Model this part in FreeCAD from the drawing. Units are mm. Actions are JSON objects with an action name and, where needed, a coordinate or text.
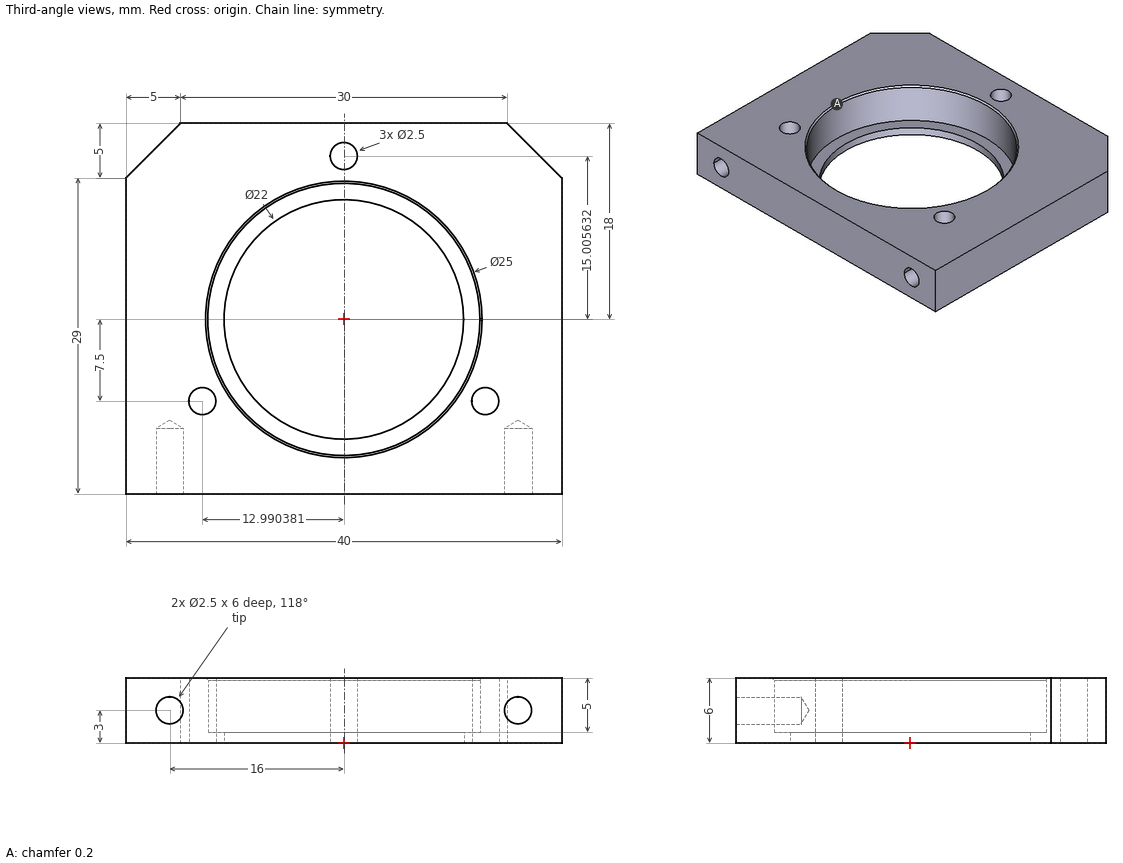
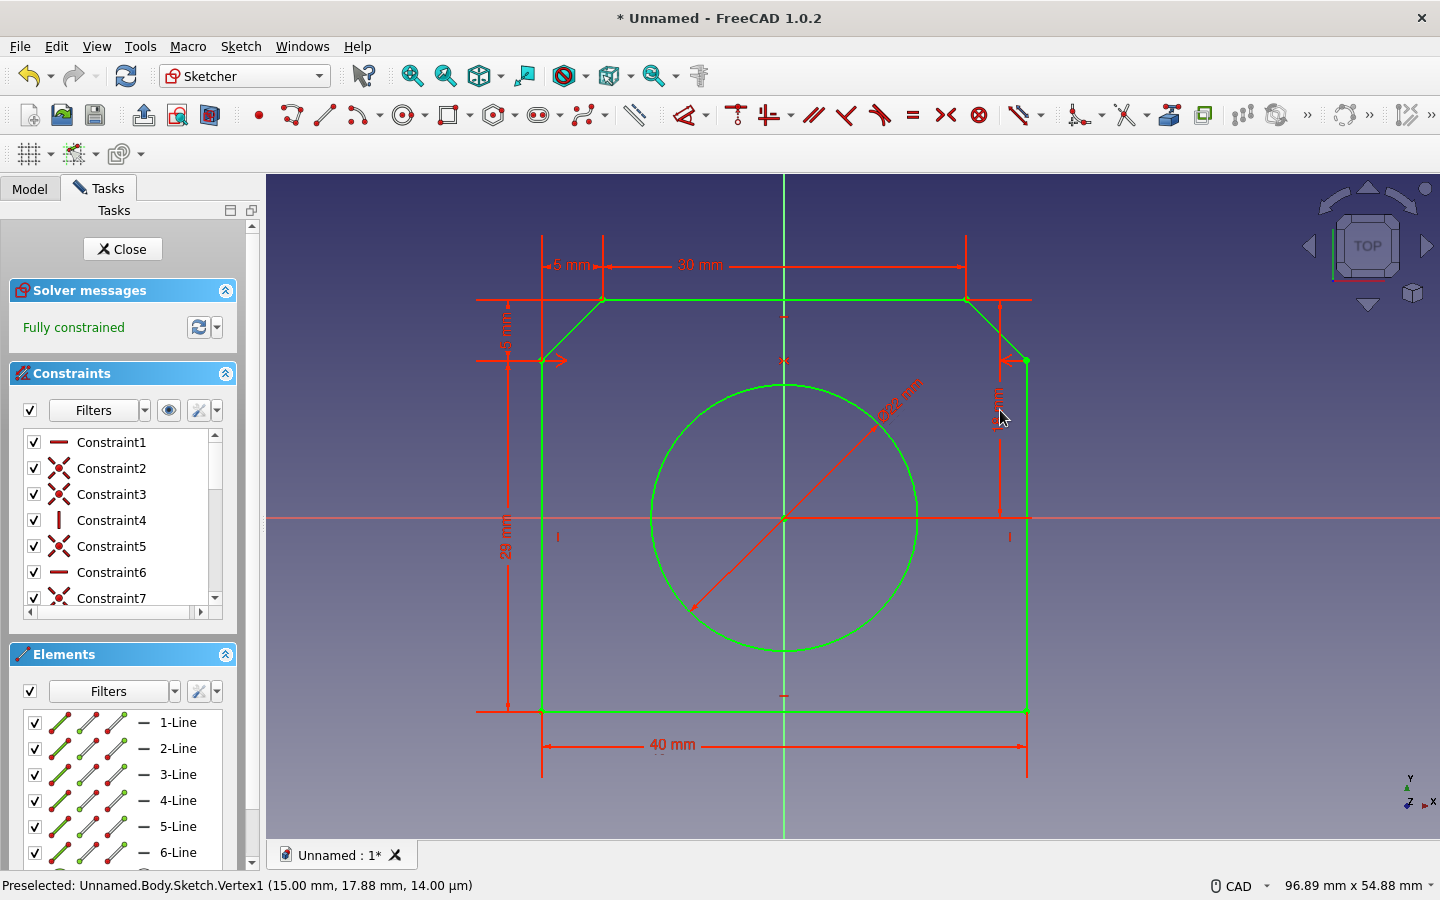
{"action": "left_click", "coordinate": [123, 249]}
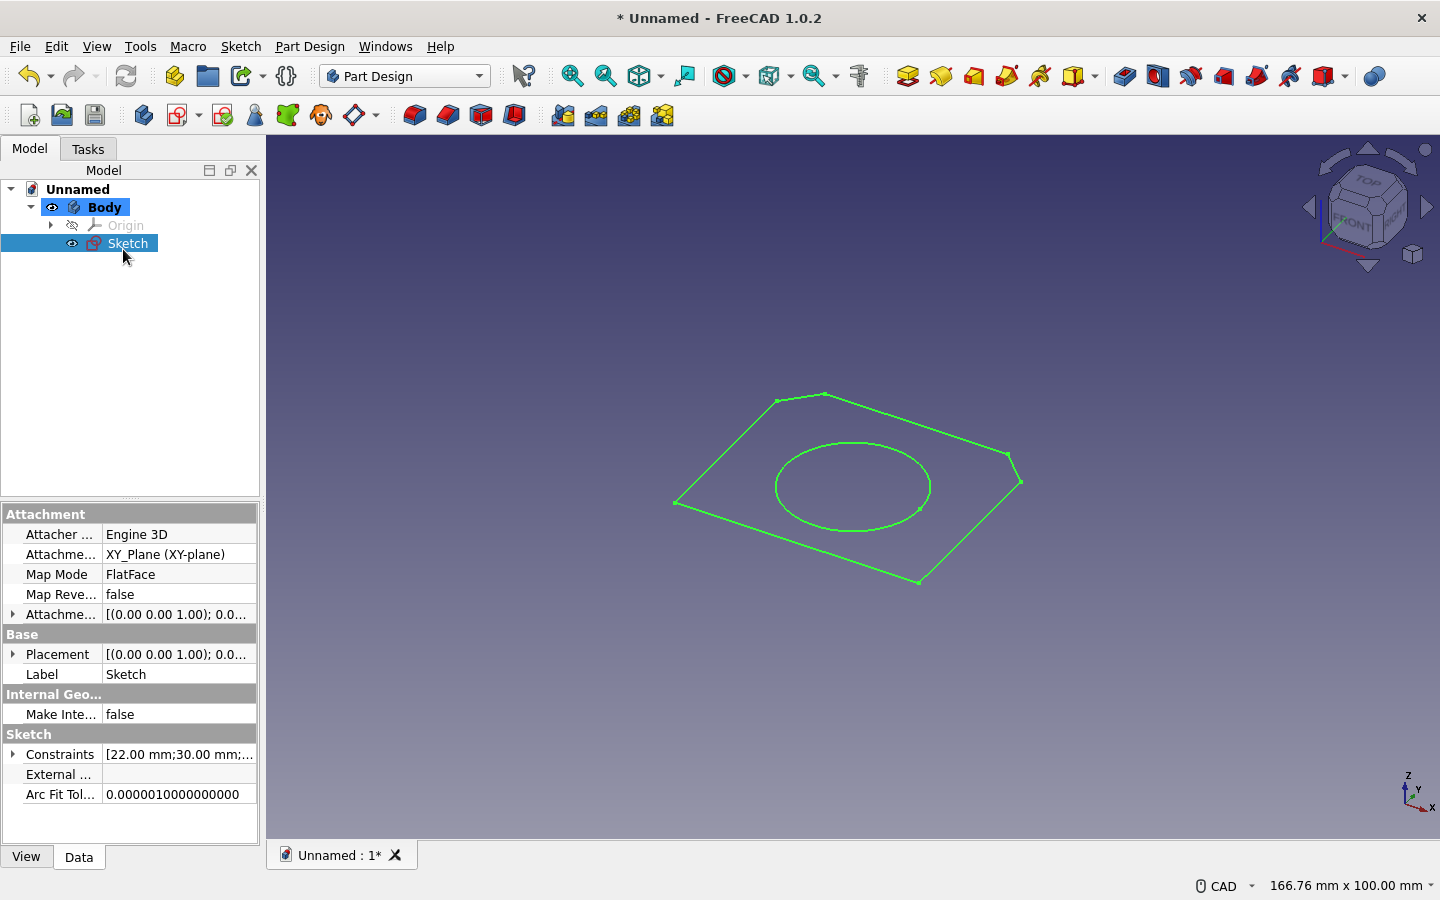
{"action": "left_click", "coordinate": [908, 76]}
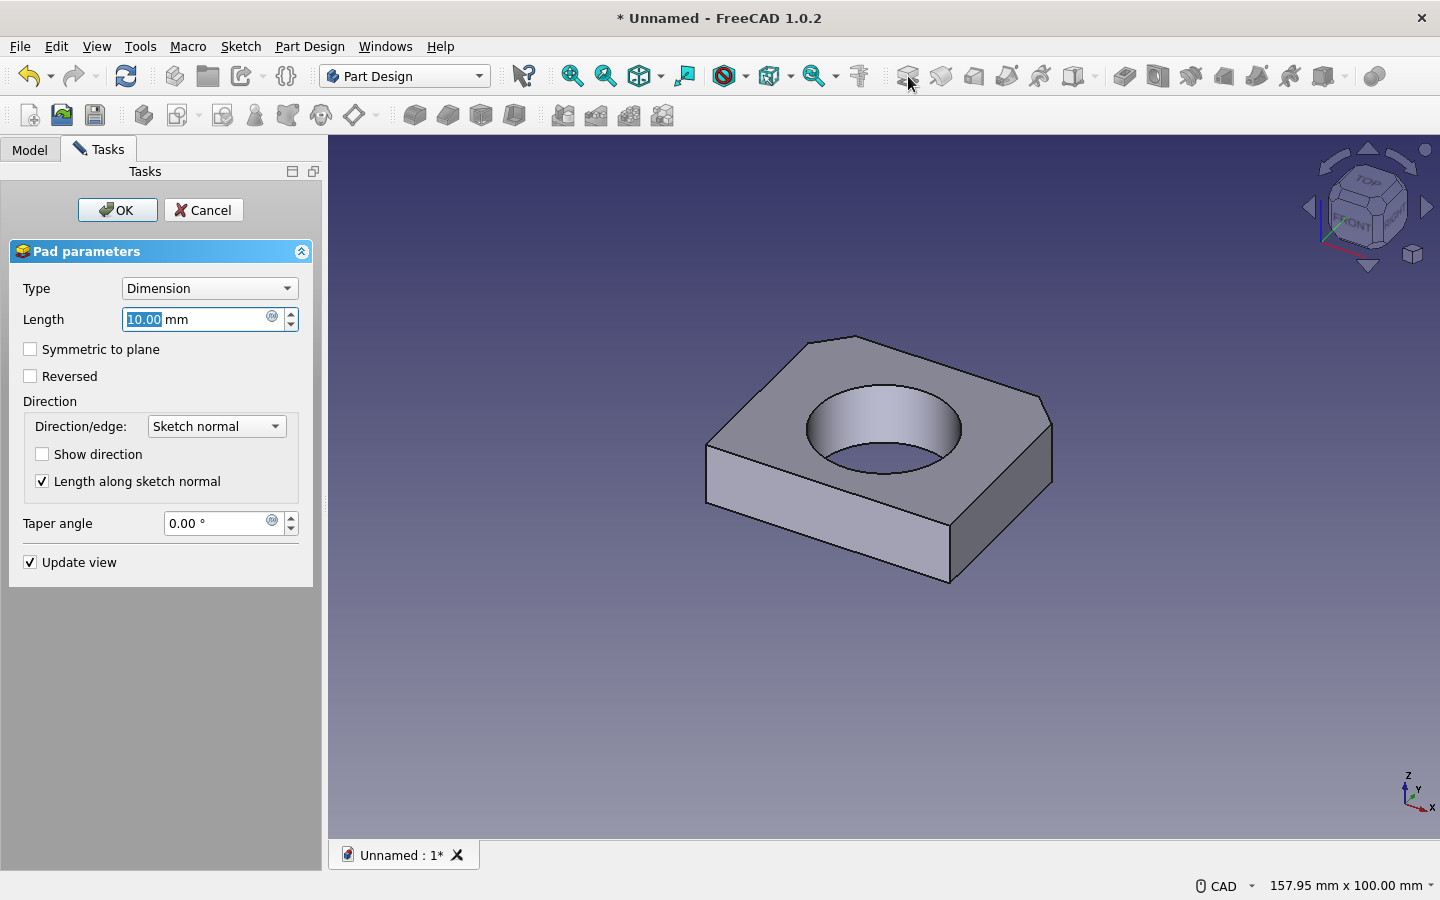
{"action": "type", "text": "6"}
{"action": "key", "text": "Tab"}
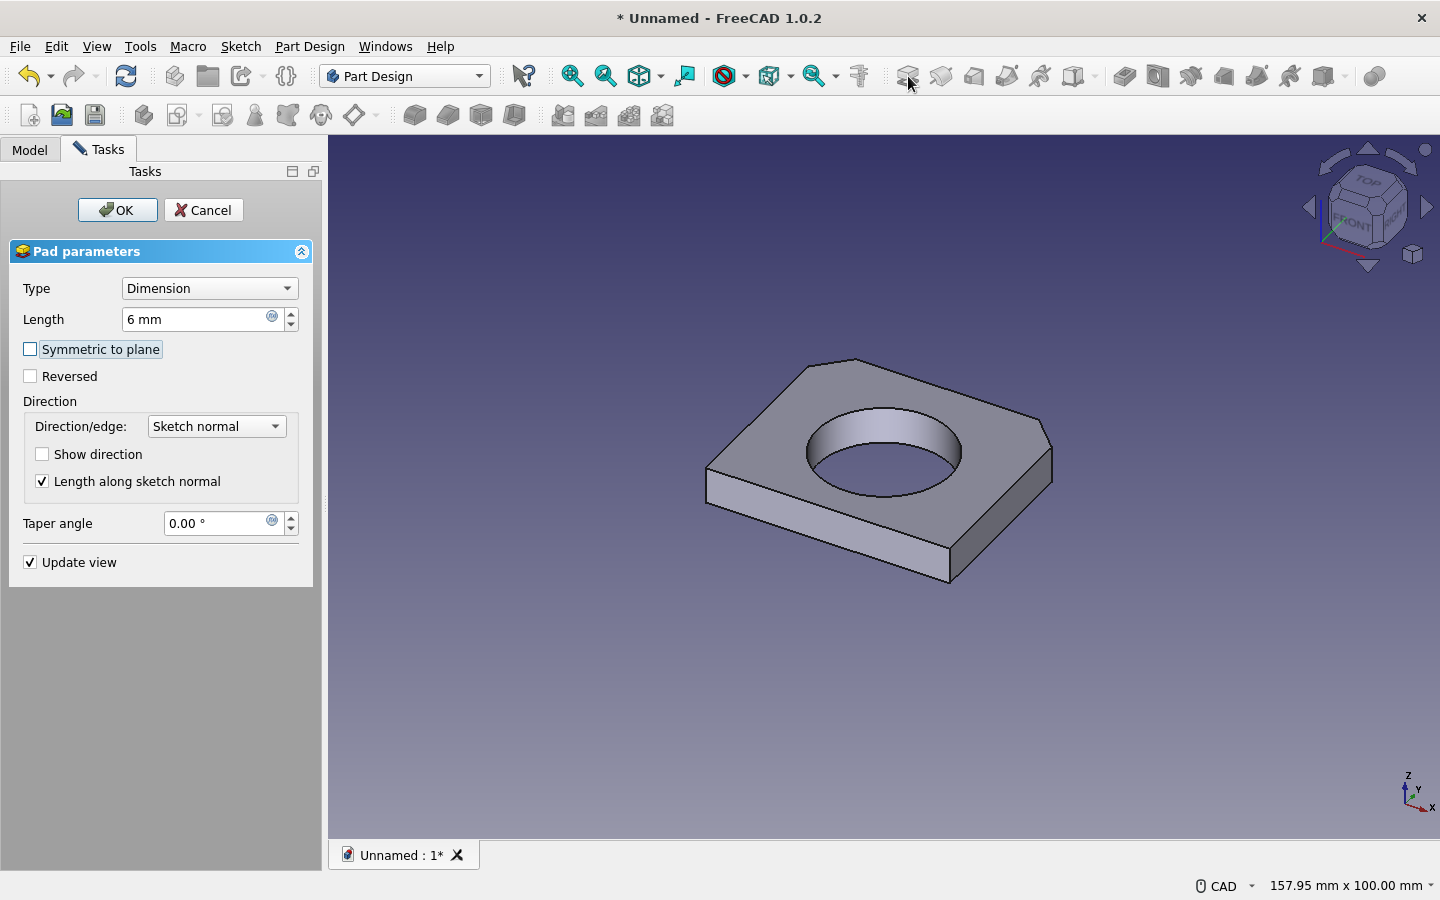
{"action": "left_click", "coordinate": [118, 210]}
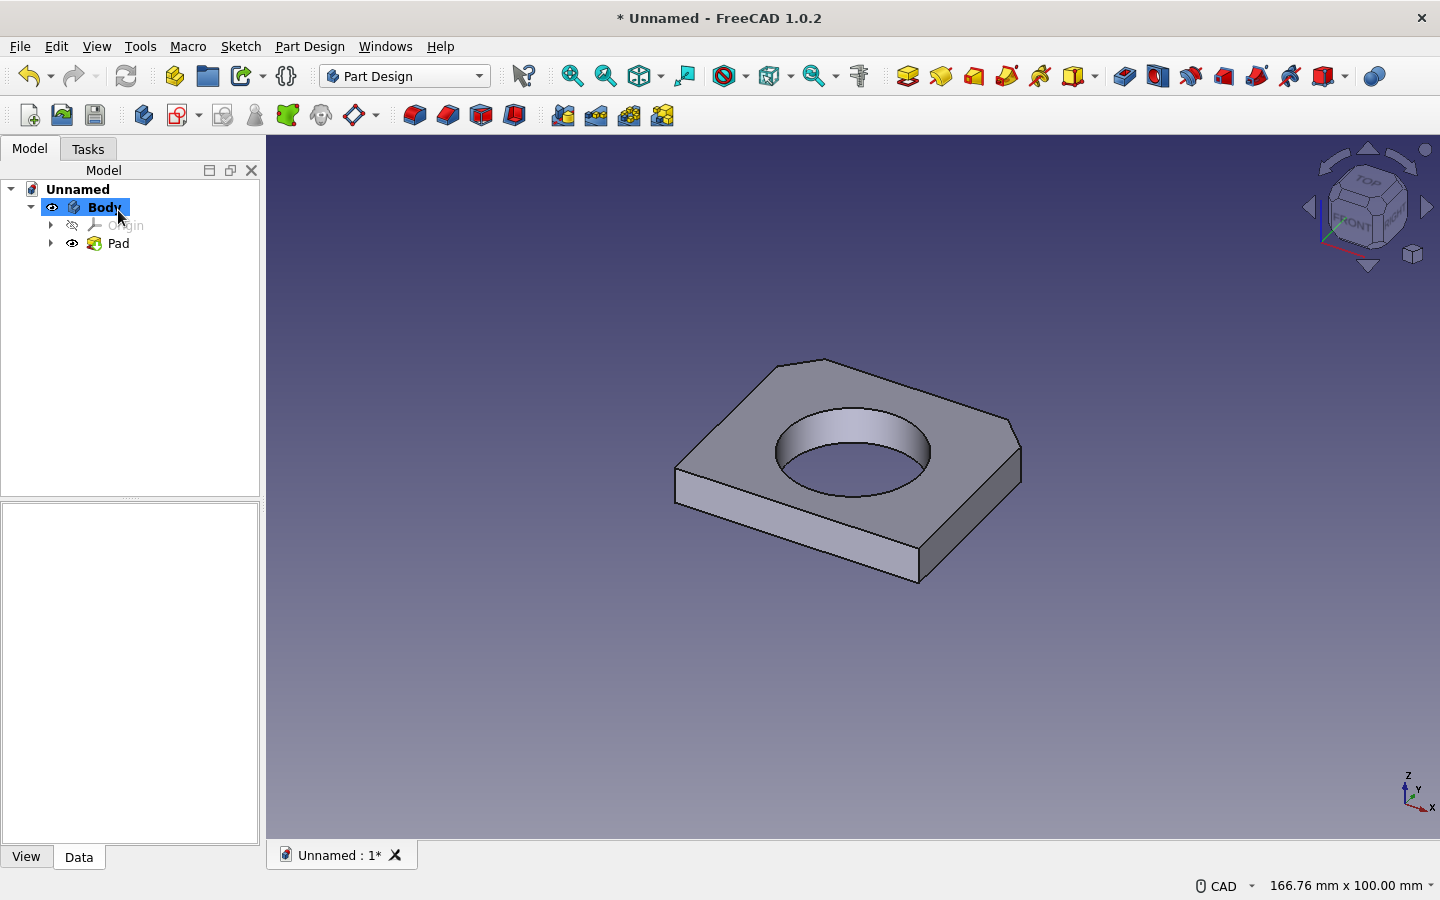
{"action": "left_click", "coordinate": [573, 76]}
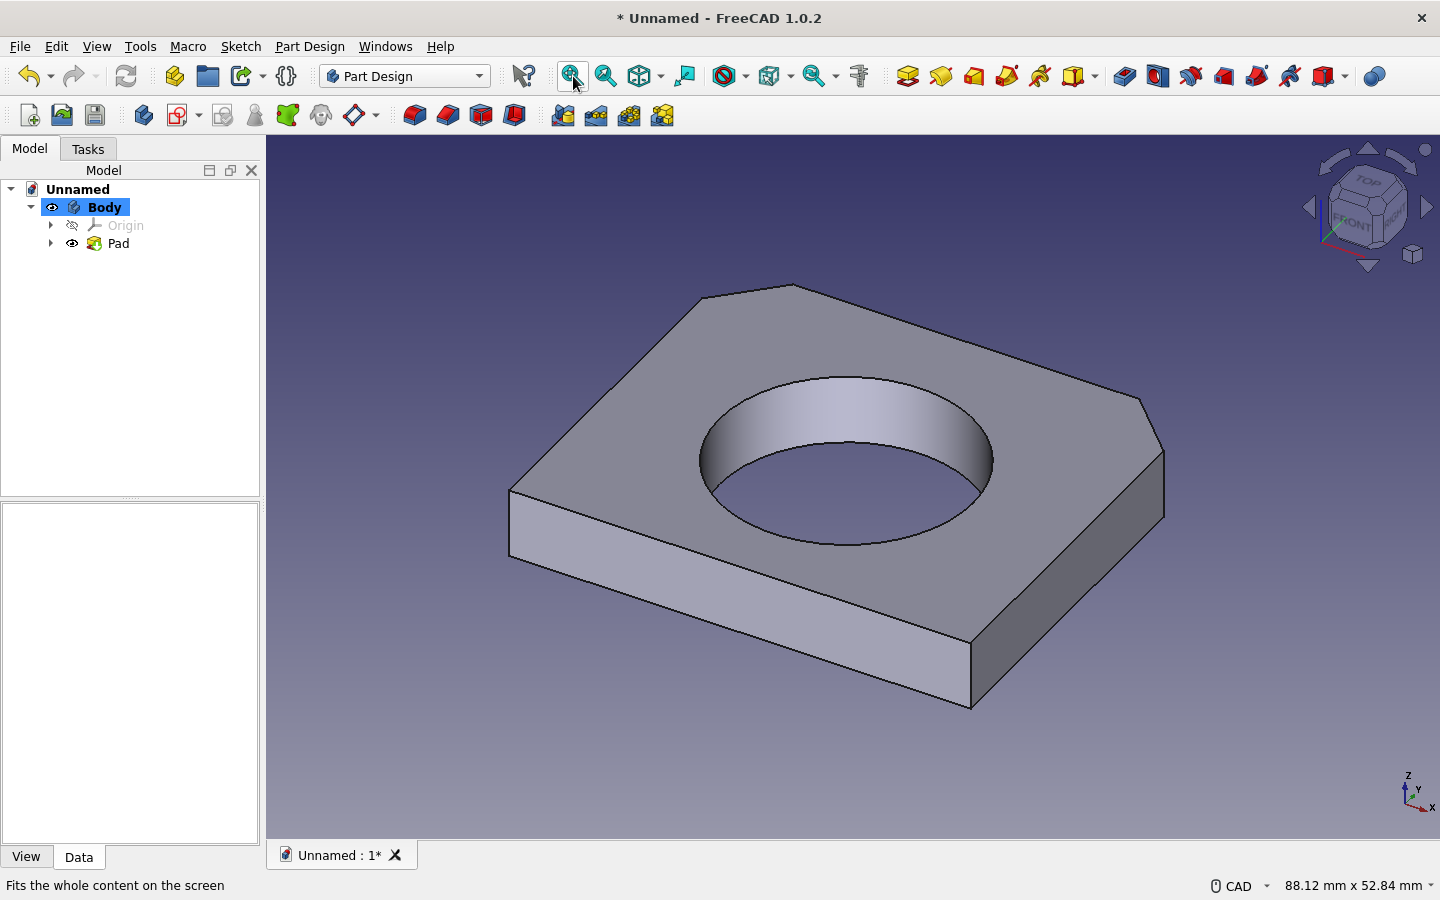
{"action": "left_click", "coordinate": [786, 345]}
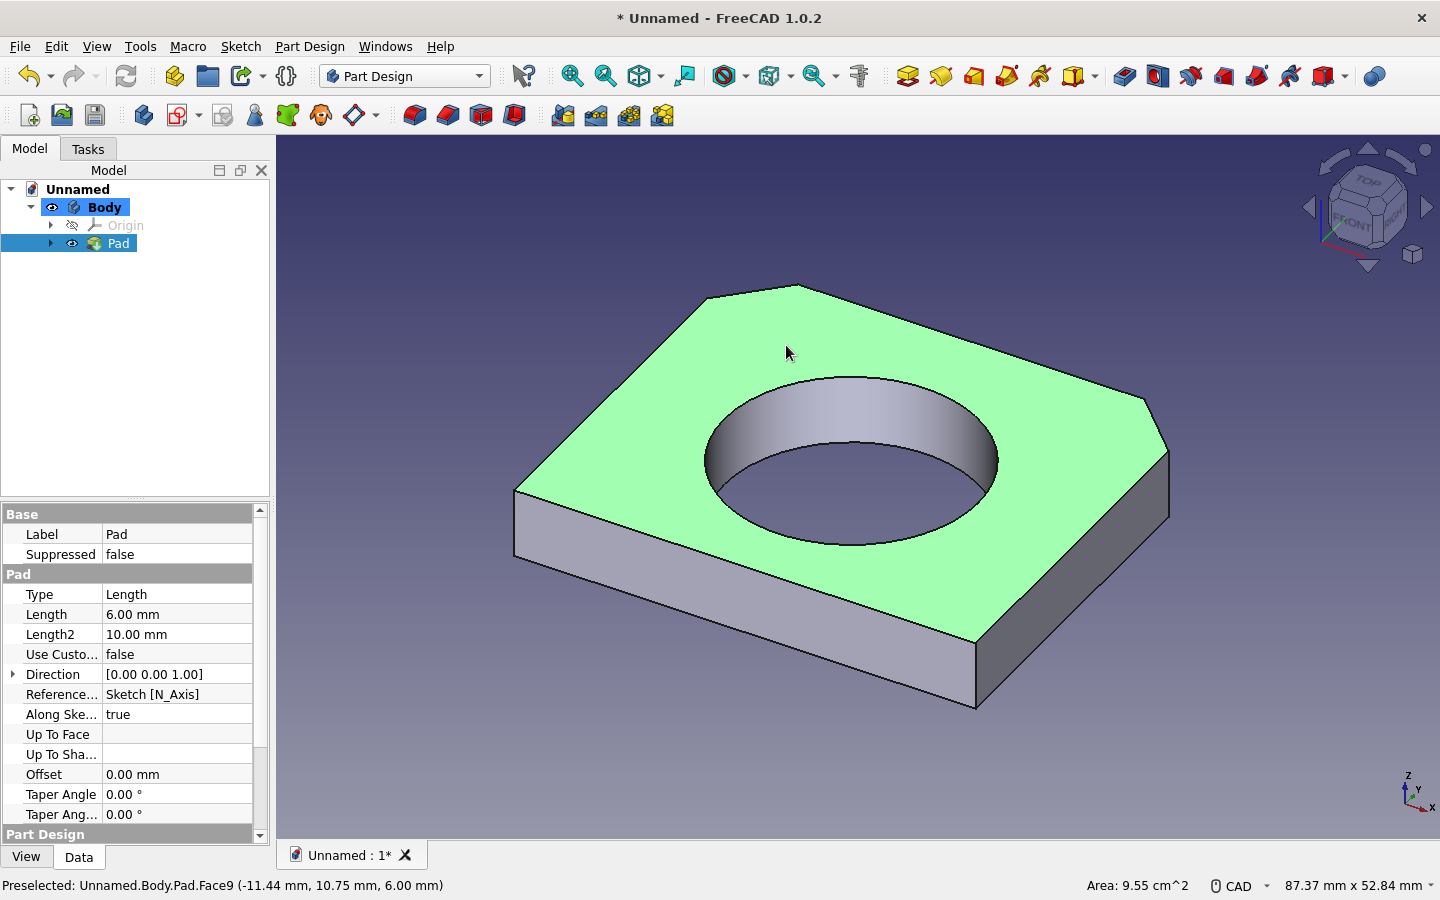
{"action": "left_click", "coordinate": [176, 116]}